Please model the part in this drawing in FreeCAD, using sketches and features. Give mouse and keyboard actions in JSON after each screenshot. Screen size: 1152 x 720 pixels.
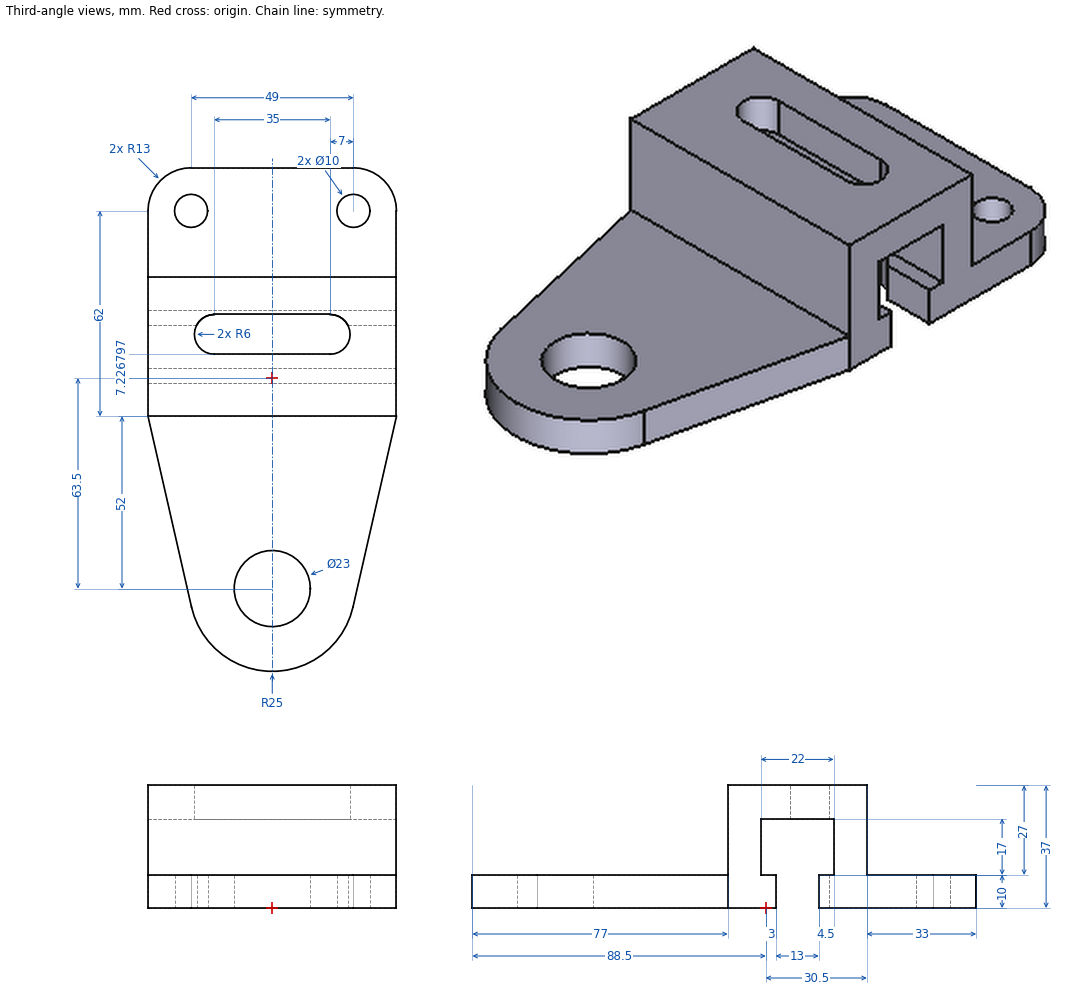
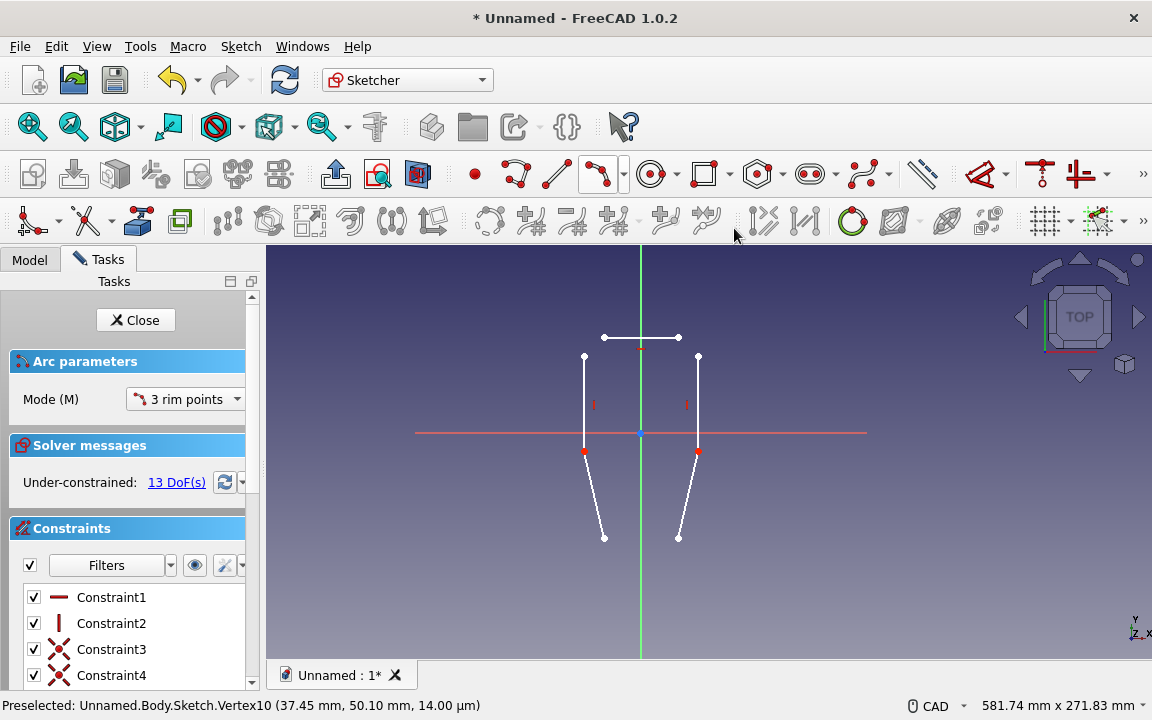
{"action": "left_click", "coordinate": [604, 338]}
{"action": "left_click", "coordinate": [584, 357]}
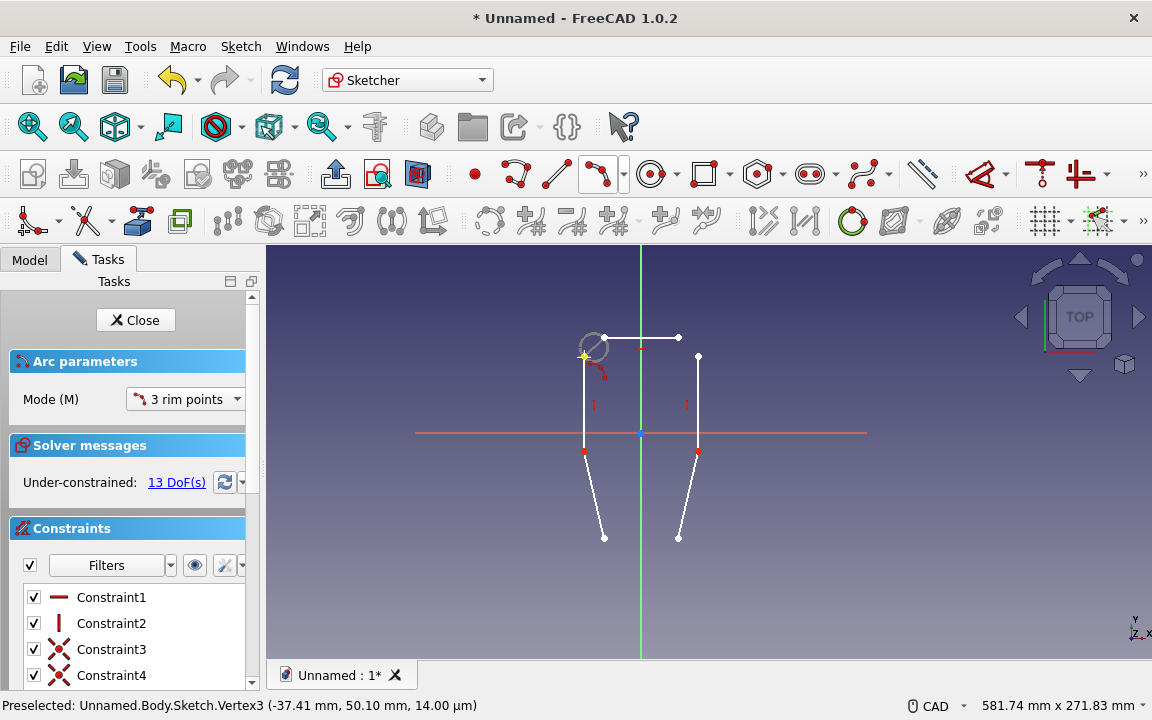
{"action": "scroll", "coordinate": [590, 342], "scroll_direction": "up", "scroll_amount": 6}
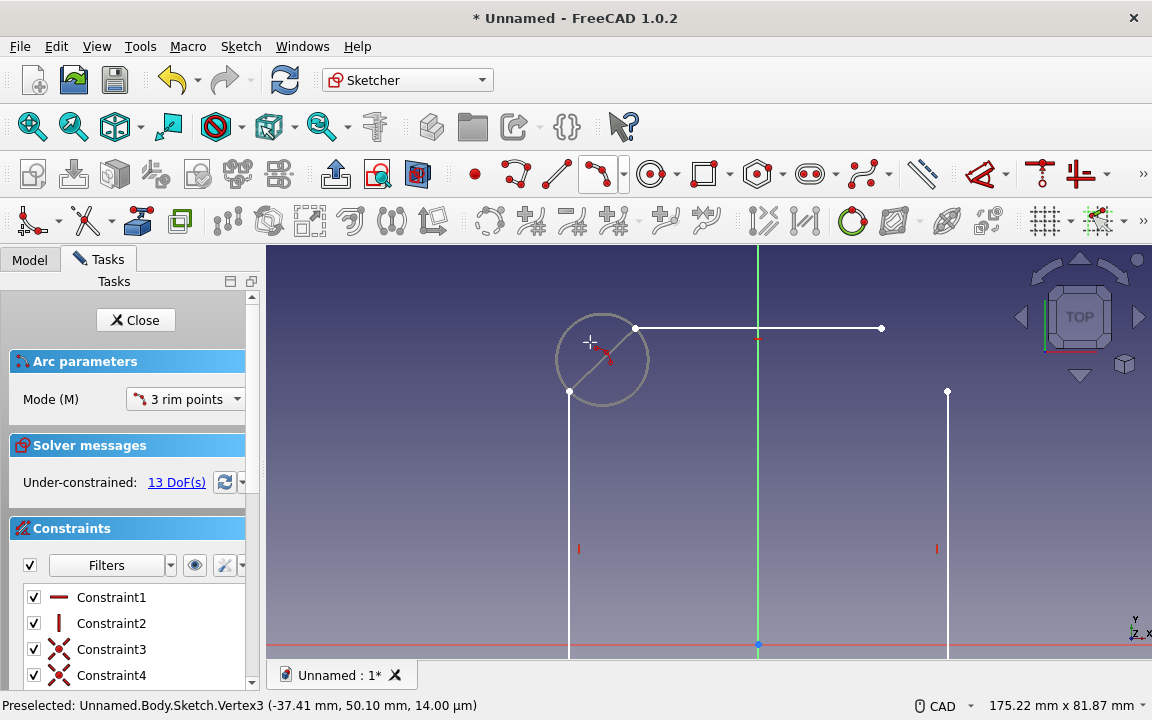
{"action": "left_click", "coordinate": [588, 343]}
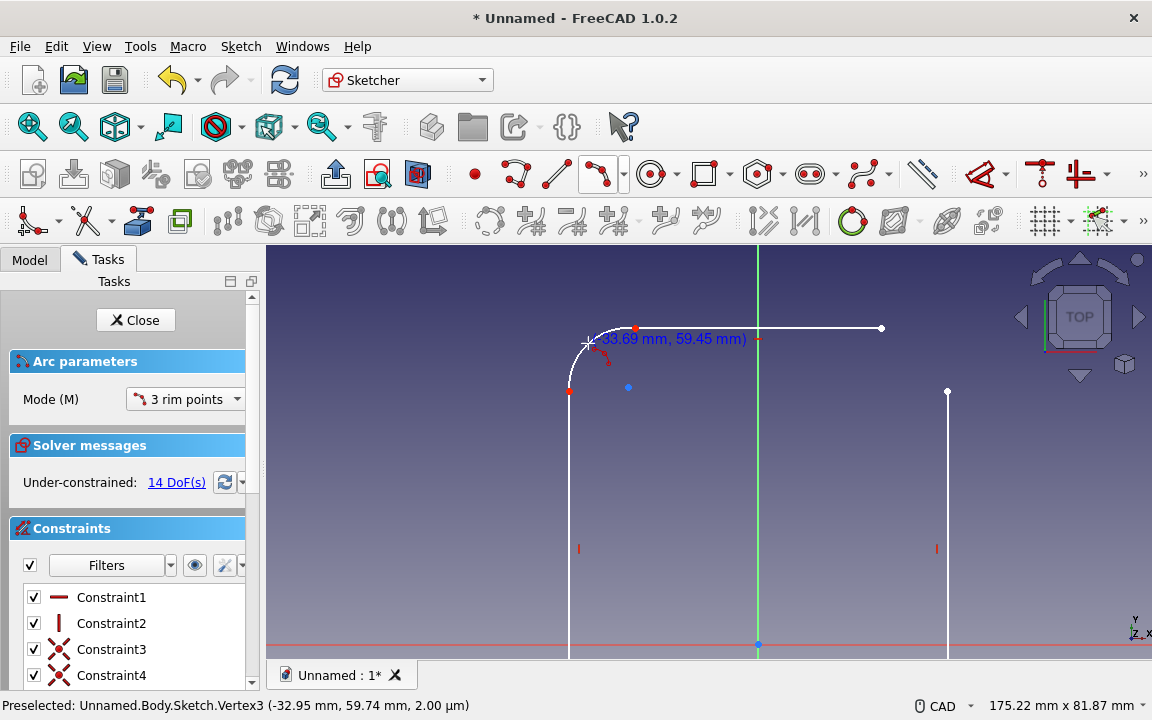
{"action": "scroll", "coordinate": [590, 342], "scroll_direction": "down", "scroll_amount": 6}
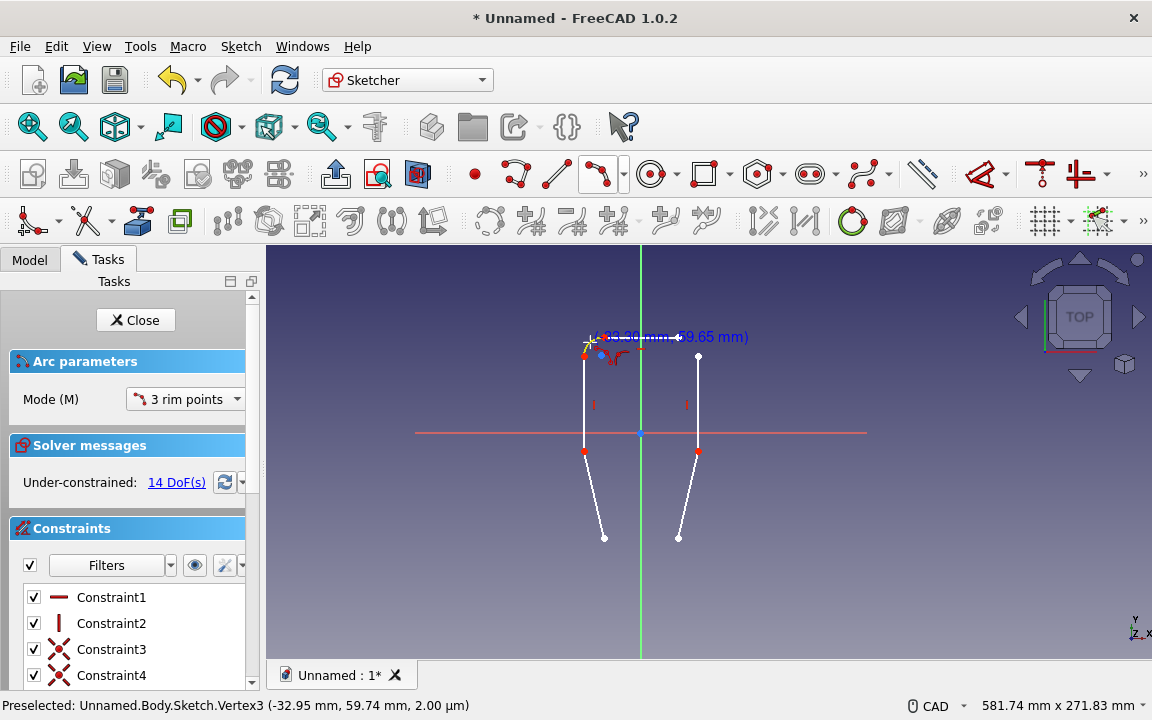
{"action": "left_click", "coordinate": [604, 539]}
{"action": "left_click", "coordinate": [678, 539]}
{"action": "left_click", "coordinate": [621, 563]}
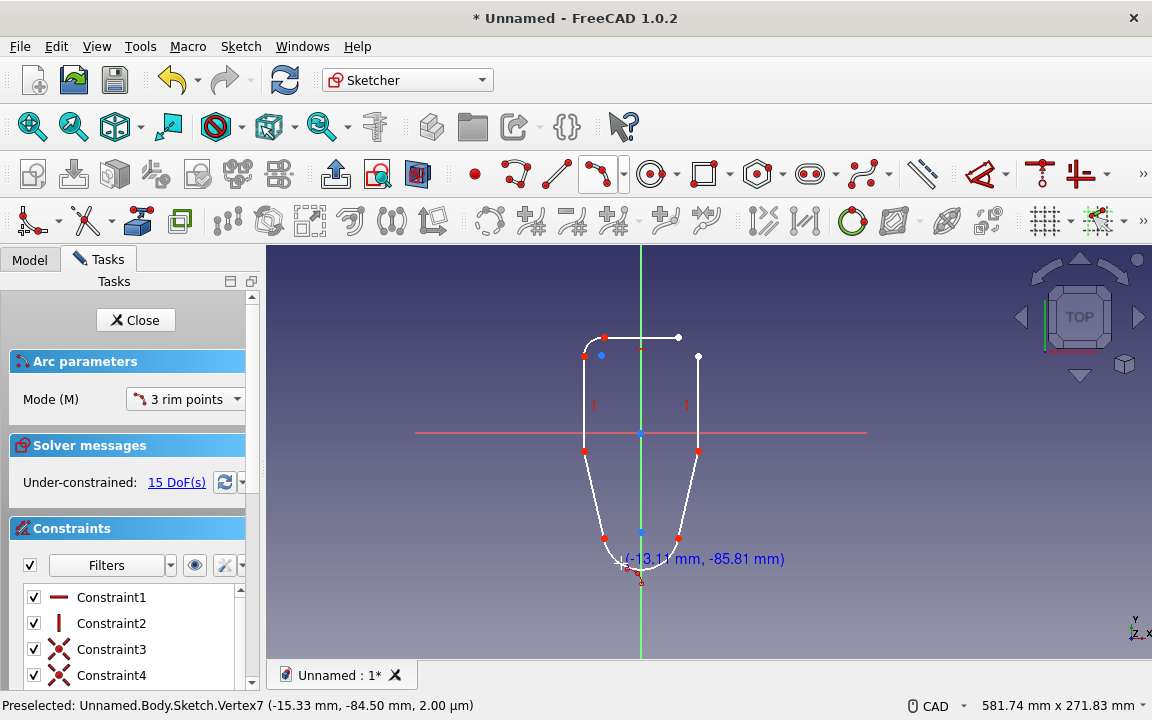
{"action": "left_click", "coordinate": [698, 357]}
{"action": "left_click", "coordinate": [678, 338]}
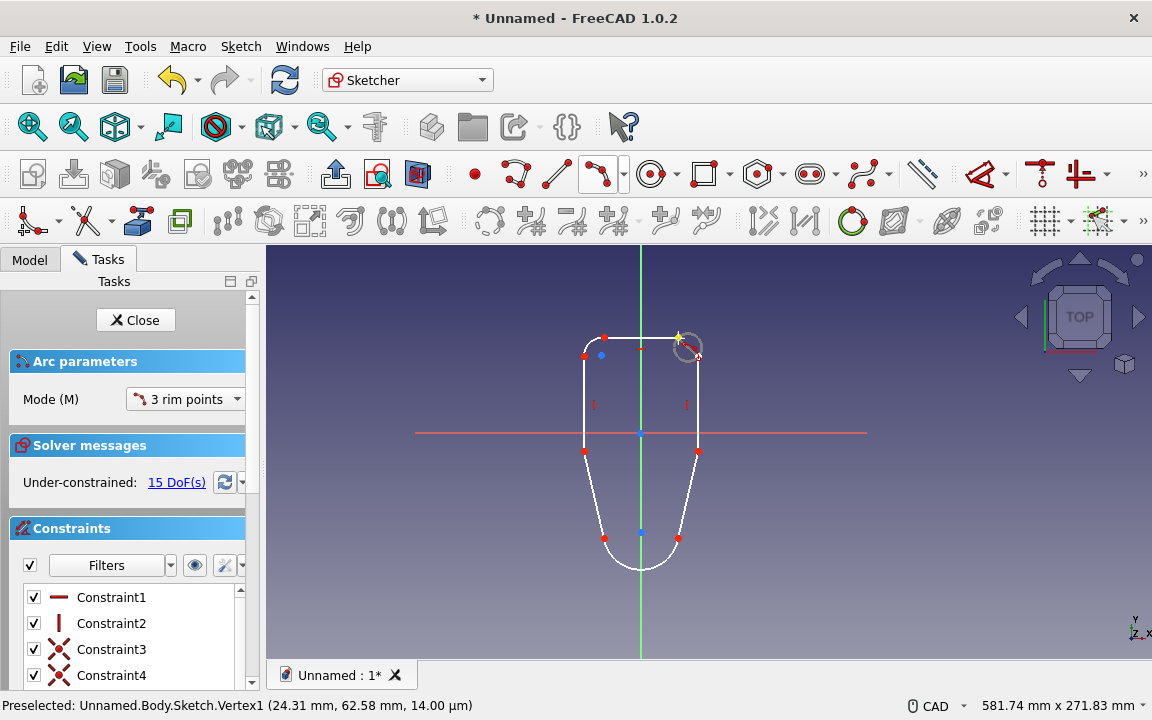
{"action": "scroll", "coordinate": [692, 342], "scroll_direction": "up", "scroll_amount": 6}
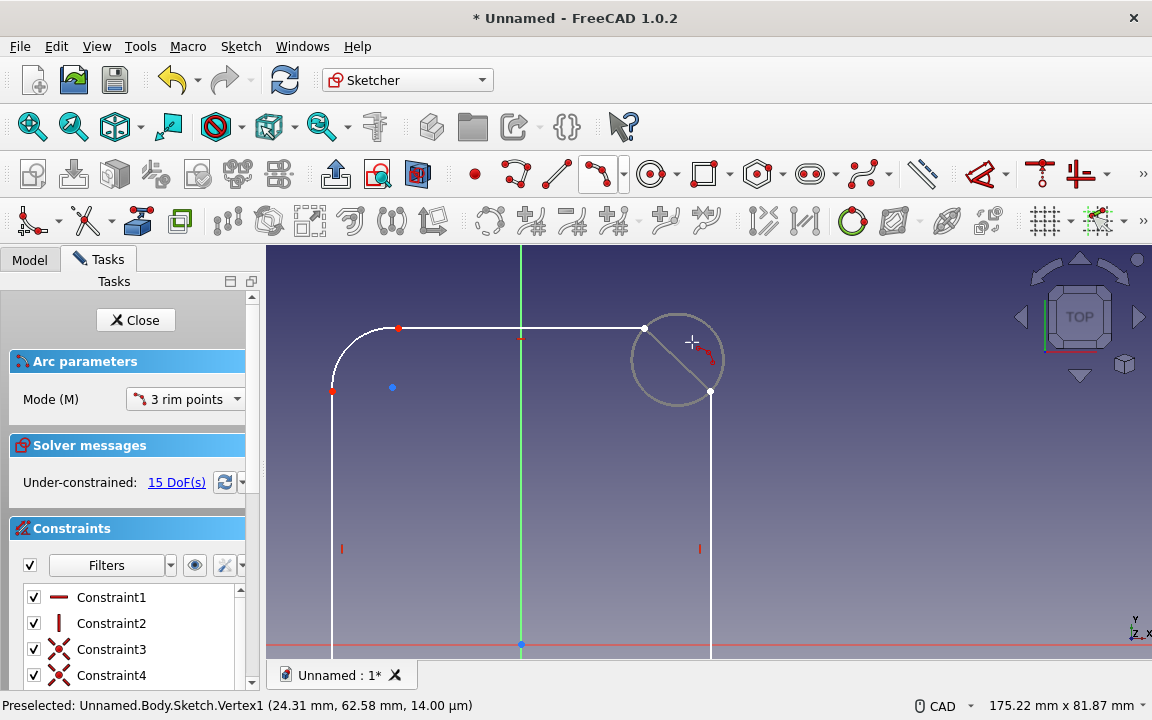
{"action": "left_click", "coordinate": [692, 343]}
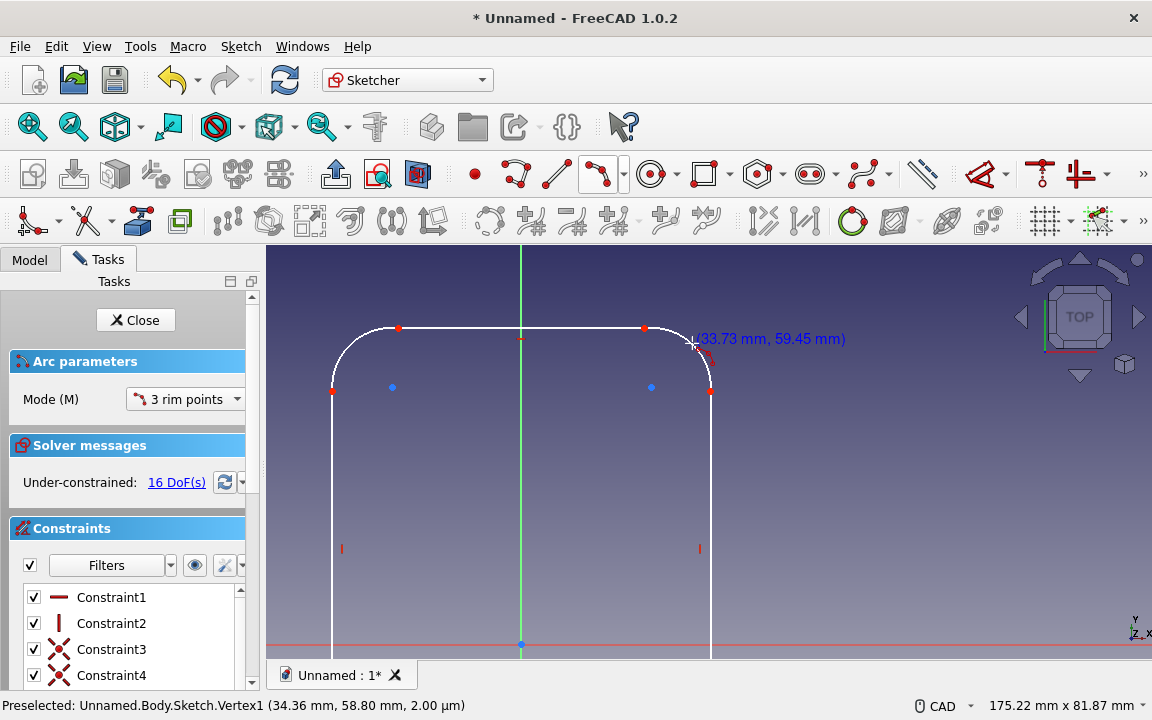
{"action": "left_click", "coordinate": [810, 174]}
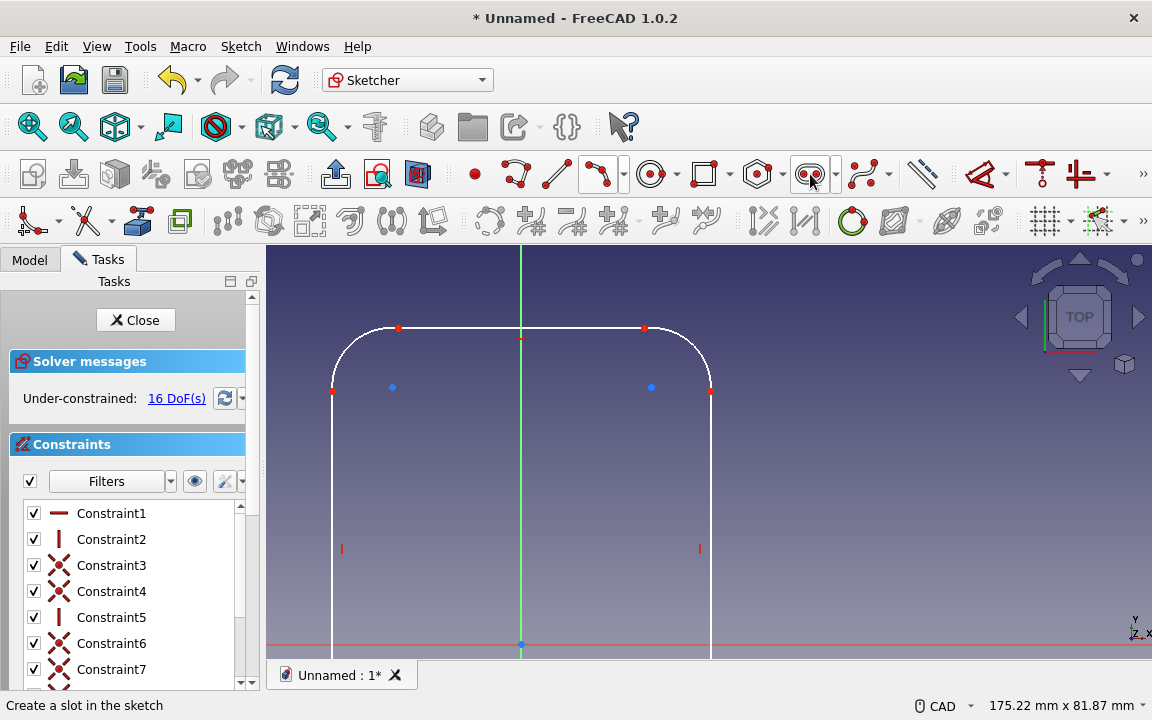
{"action": "left_click", "coordinate": [433, 578]}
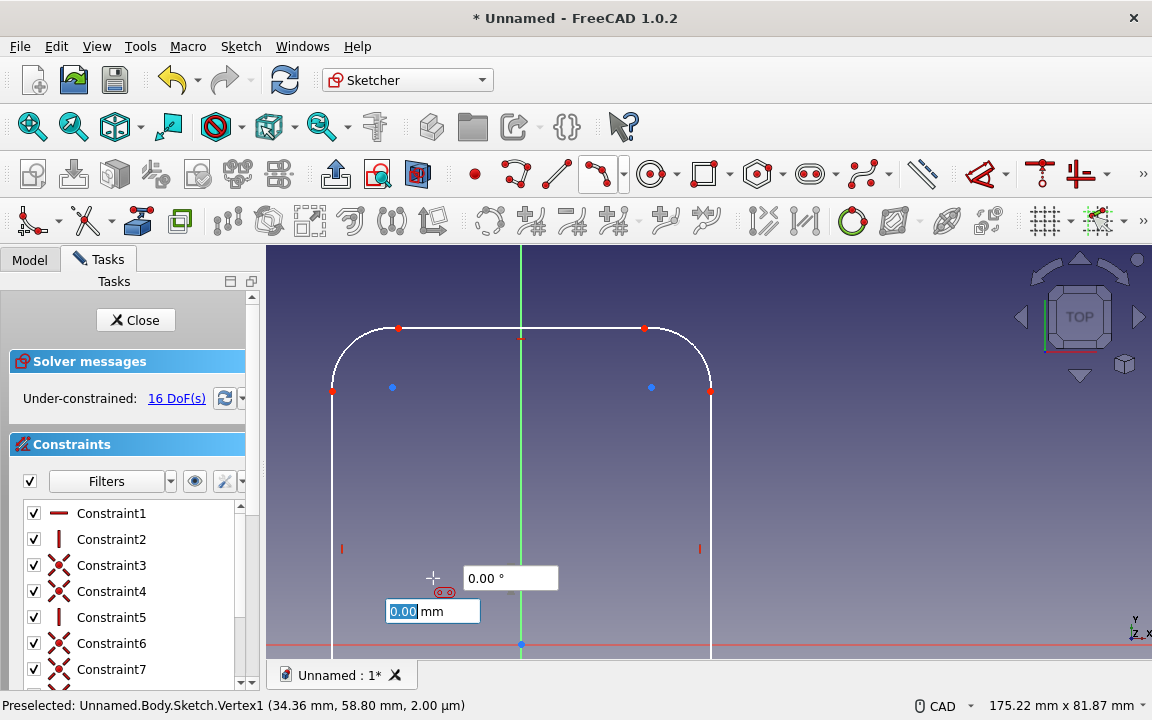
{"action": "left_click", "coordinate": [610, 578]}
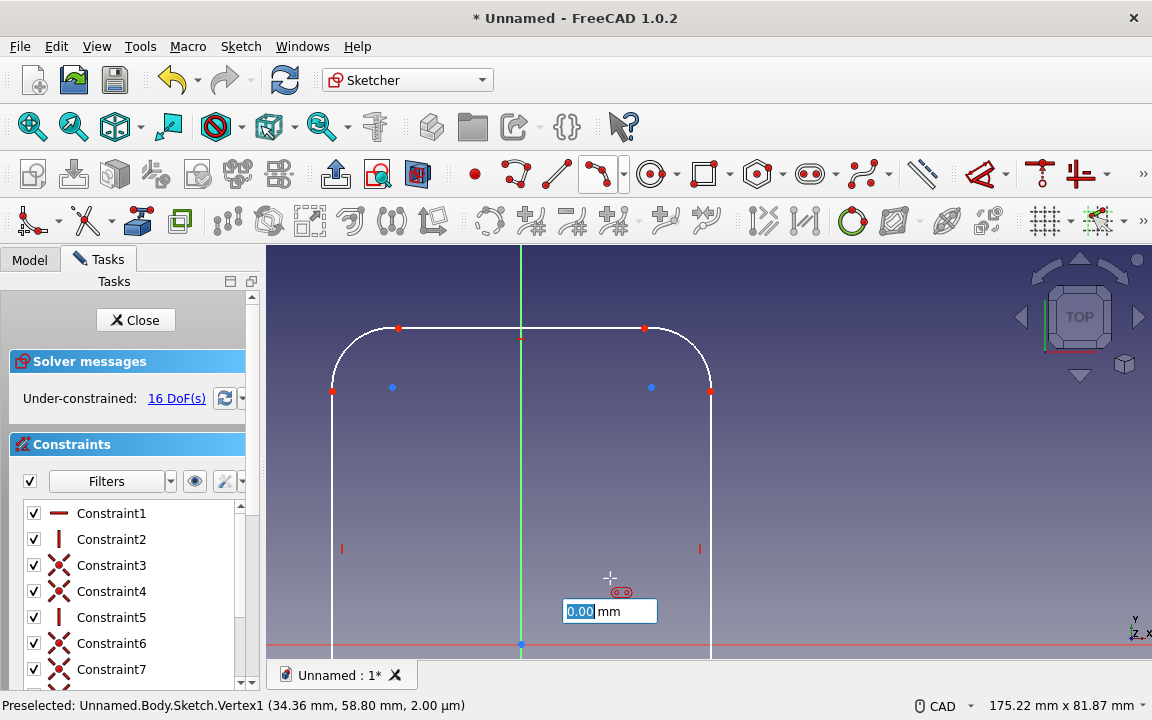
{"action": "left_click", "coordinate": [548, 608]}